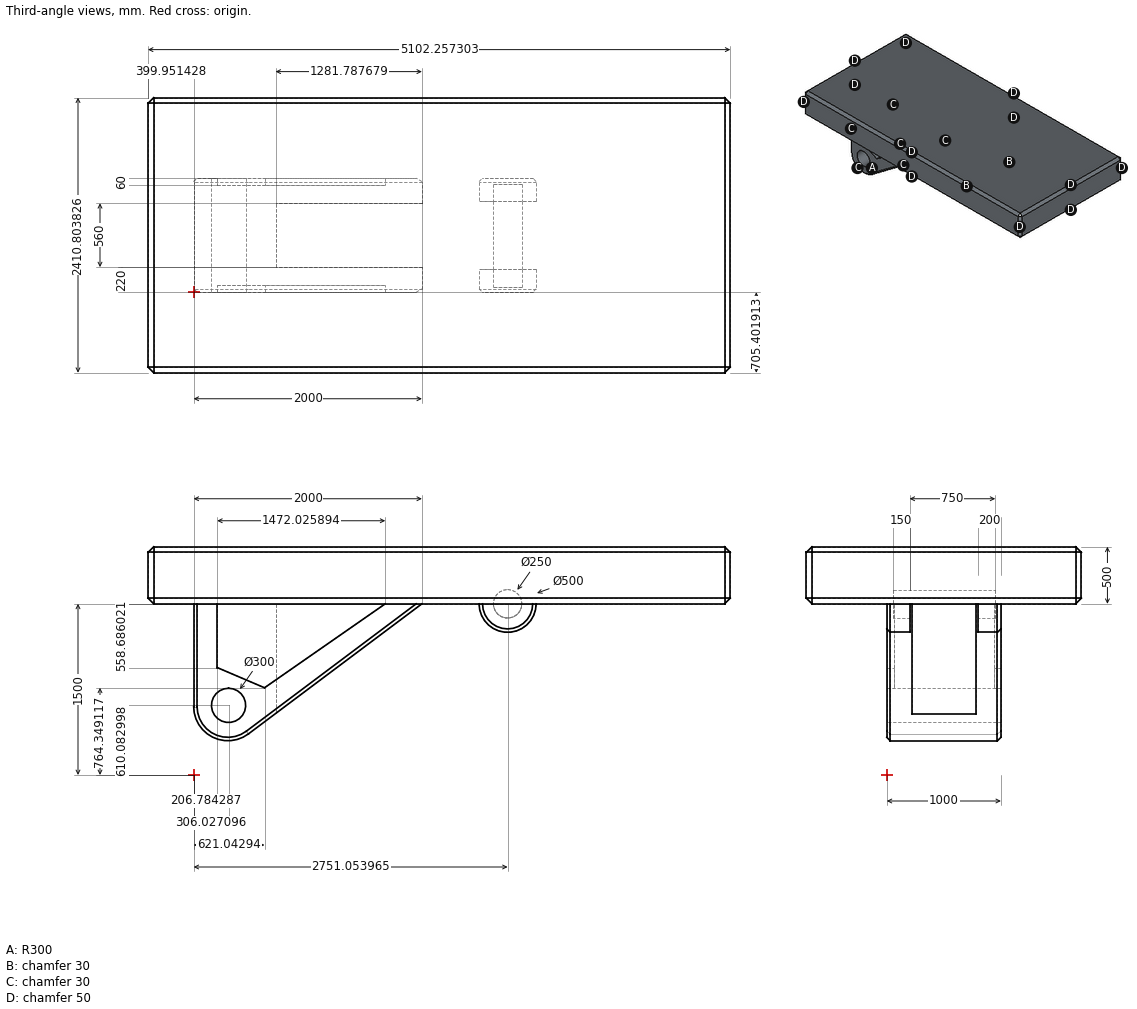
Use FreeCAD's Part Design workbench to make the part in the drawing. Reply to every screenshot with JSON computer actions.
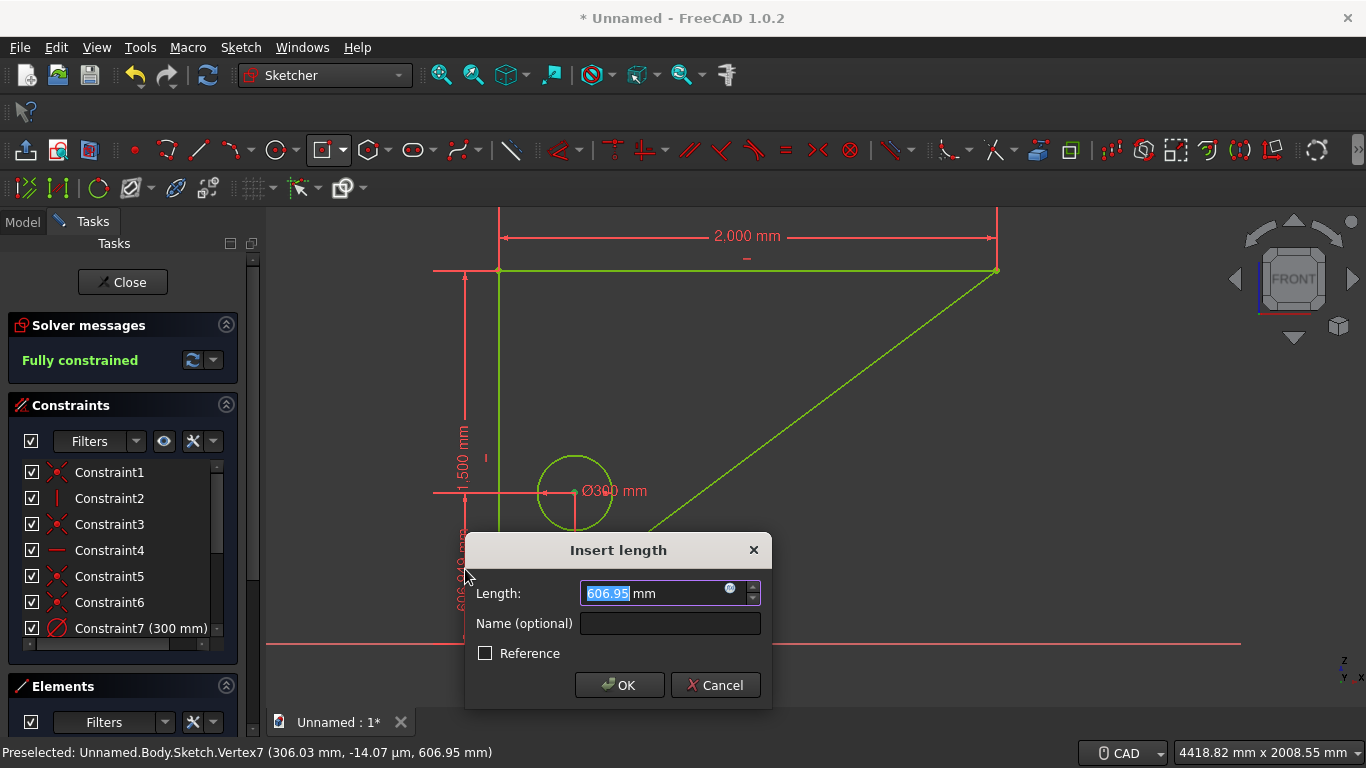
{"action": "type", "text": "610.082998"}
{"action": "key", "text": "Return"}
{"action": "key", "text": "Escape"}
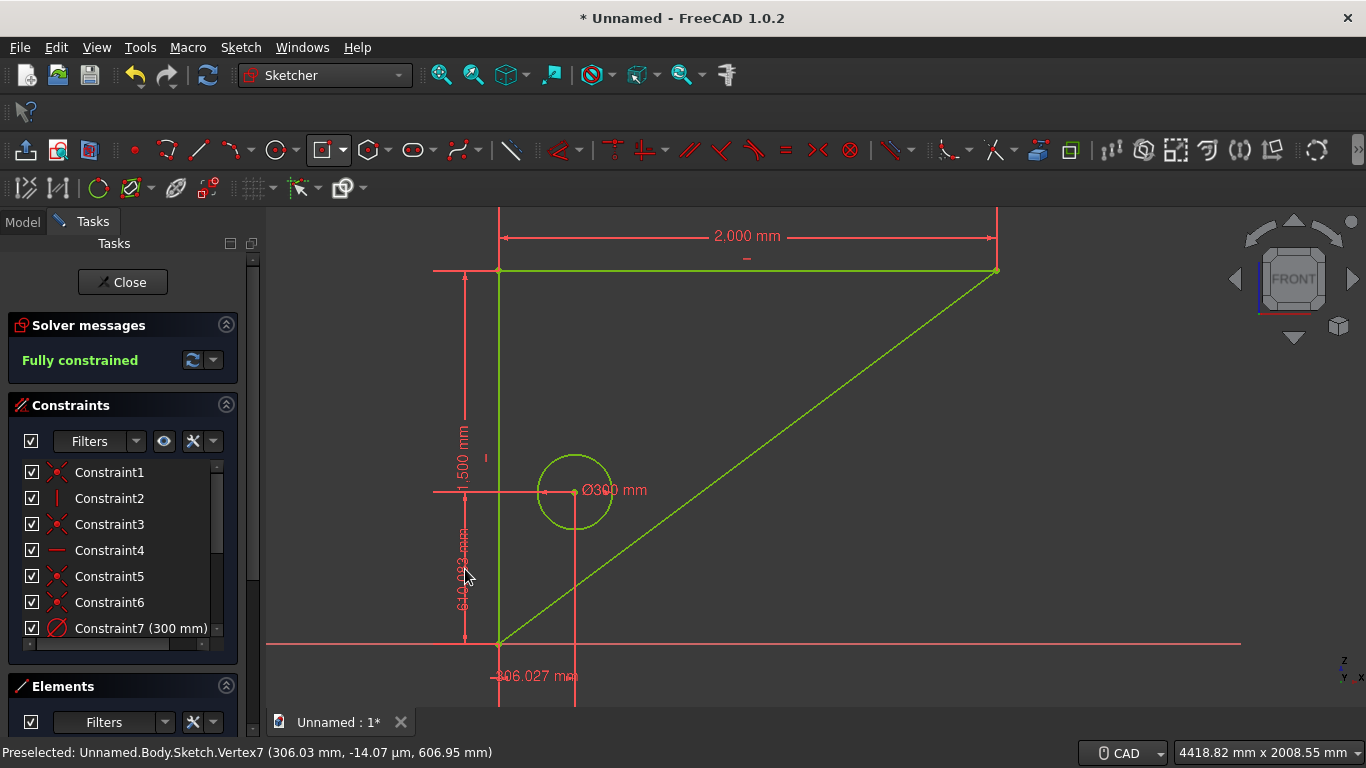
{"action": "left_click", "coordinate": [123, 282]}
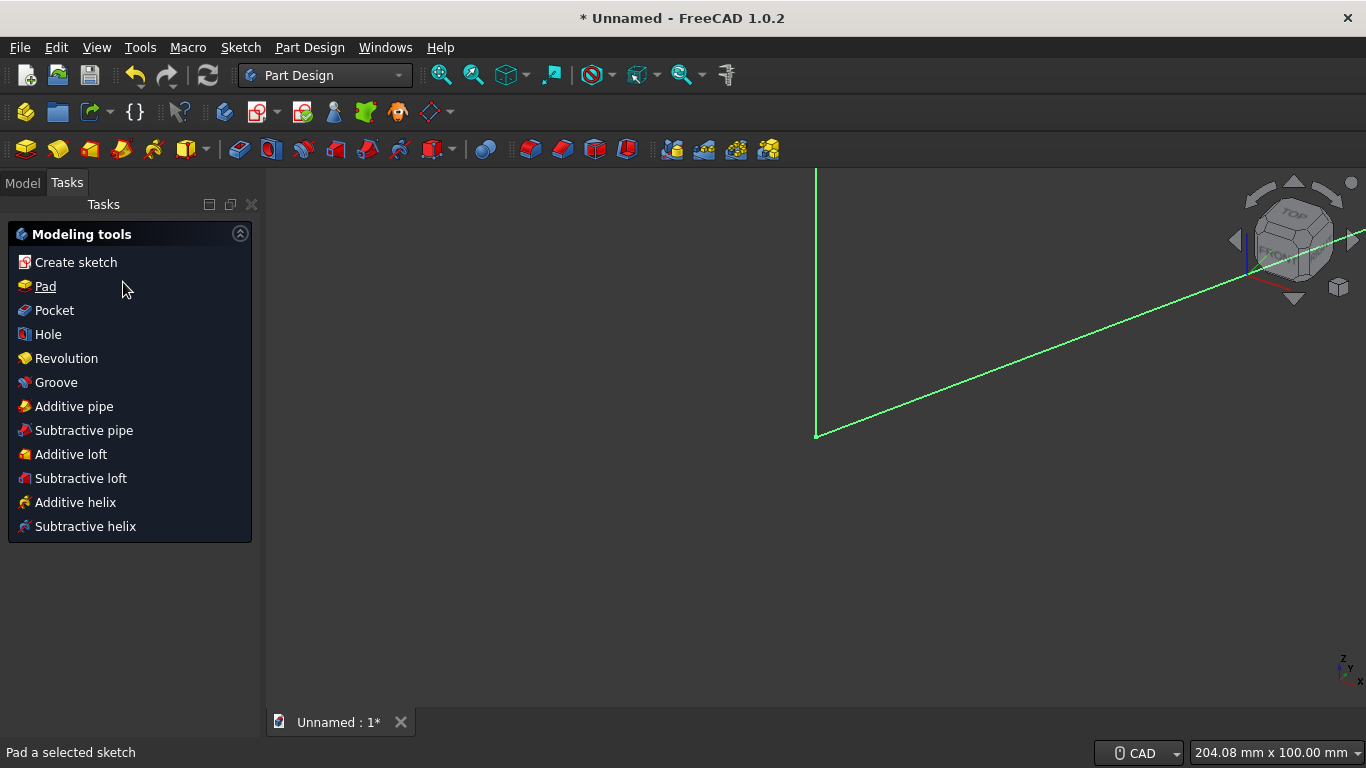
{"action": "left_click", "coordinate": [26, 150]}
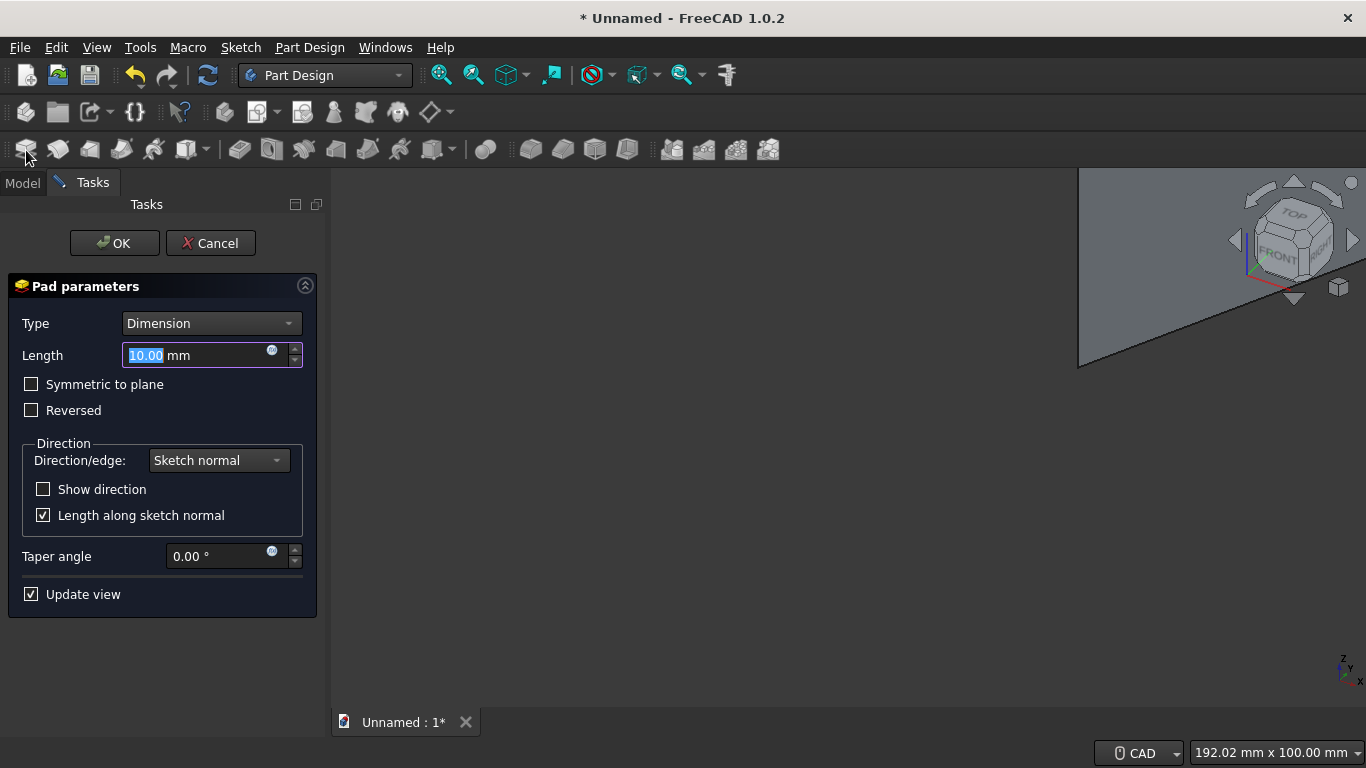
{"action": "type", "text": "1000"}
{"action": "key", "text": "Tab"}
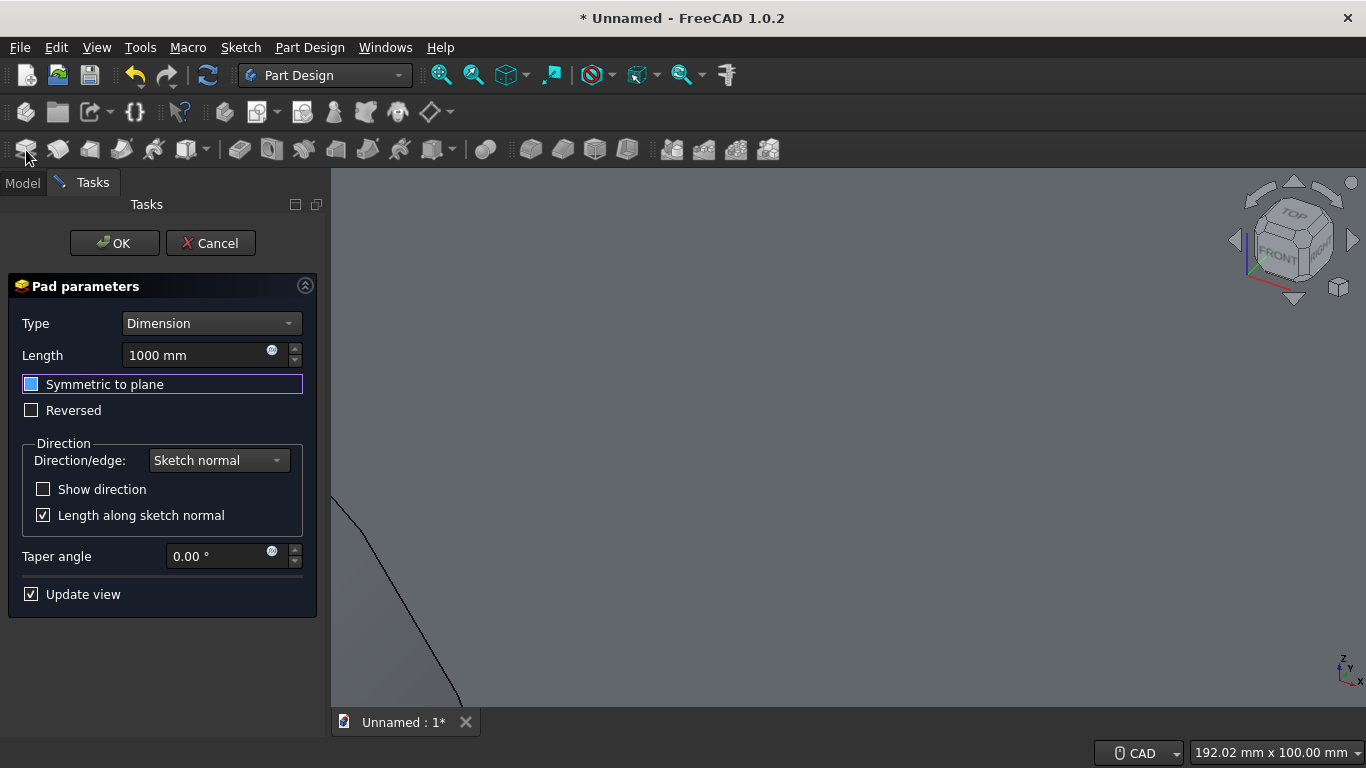
{"action": "left_click", "coordinate": [30, 410]}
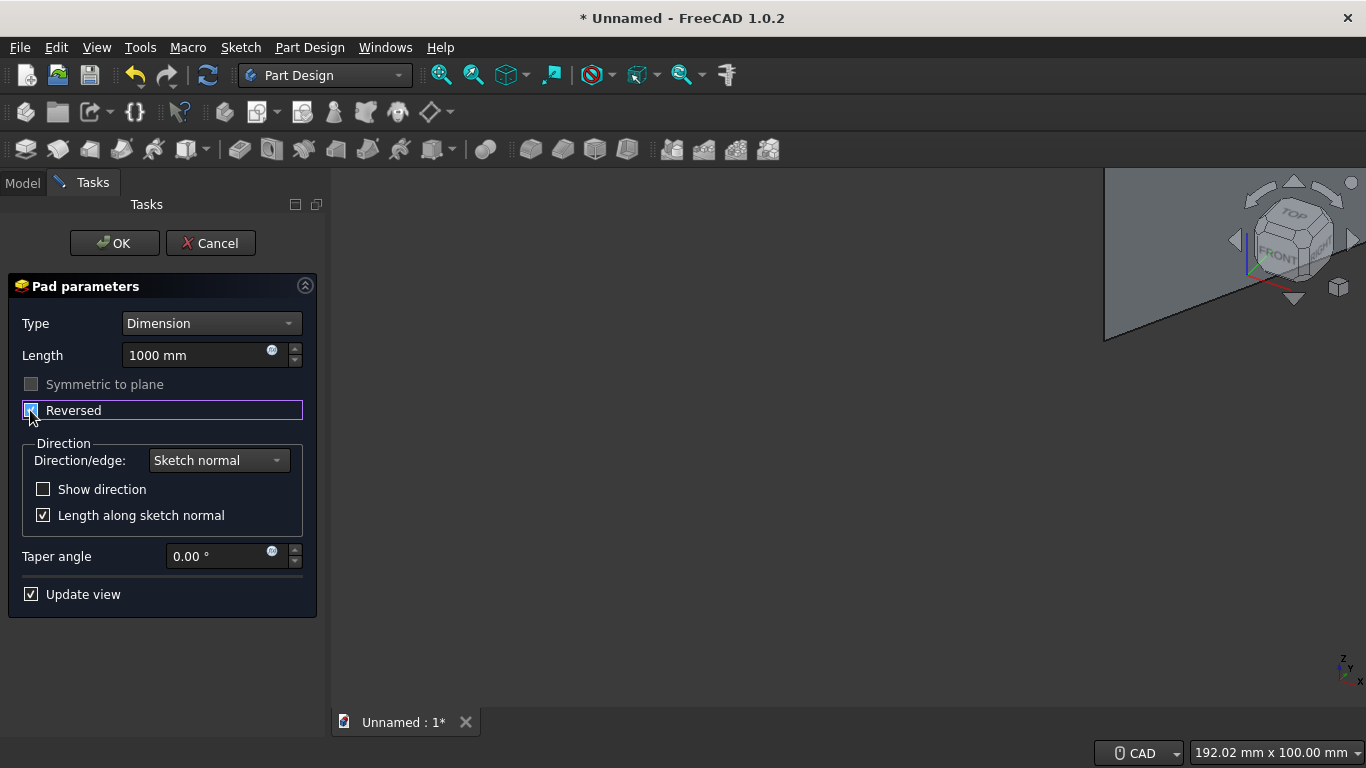
{"action": "left_click", "coordinate": [115, 243]}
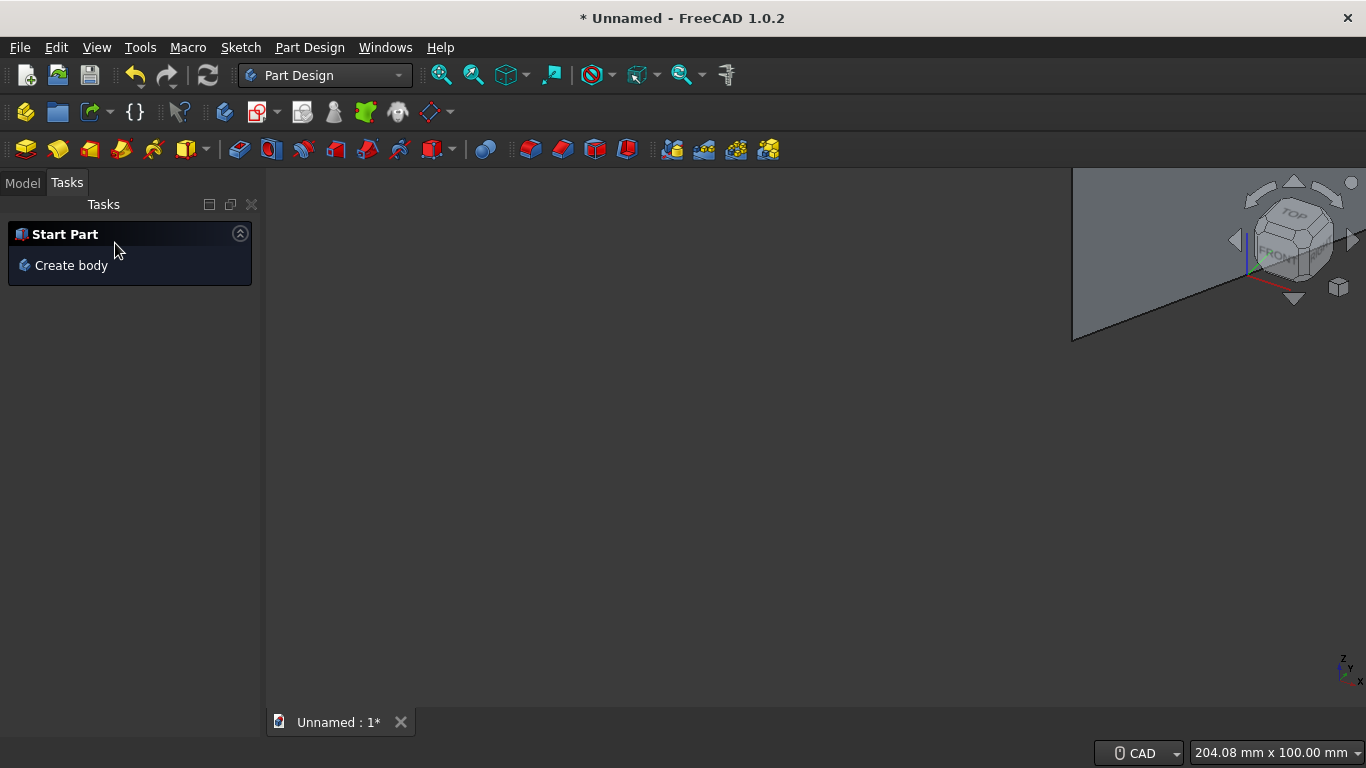
{"action": "left_click", "coordinate": [442, 76]}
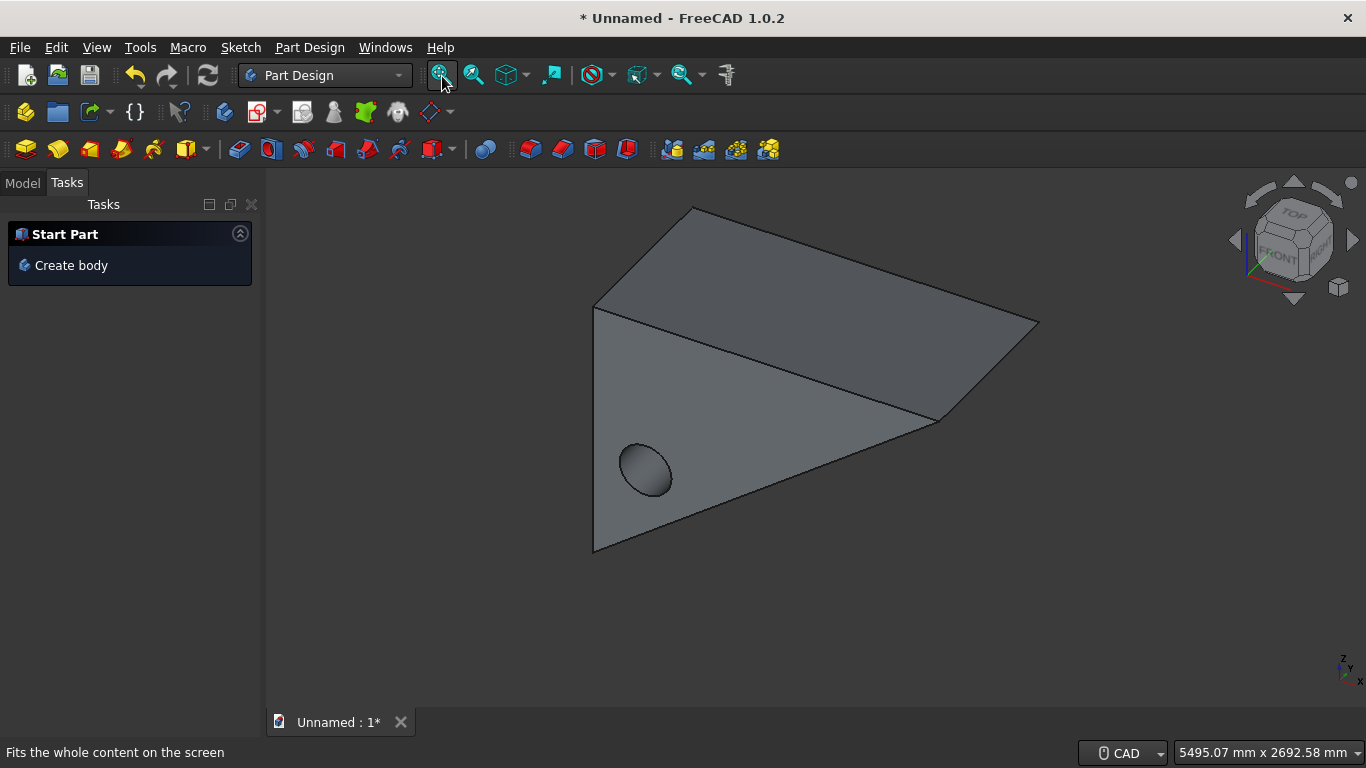
{"action": "key", "text": "0"}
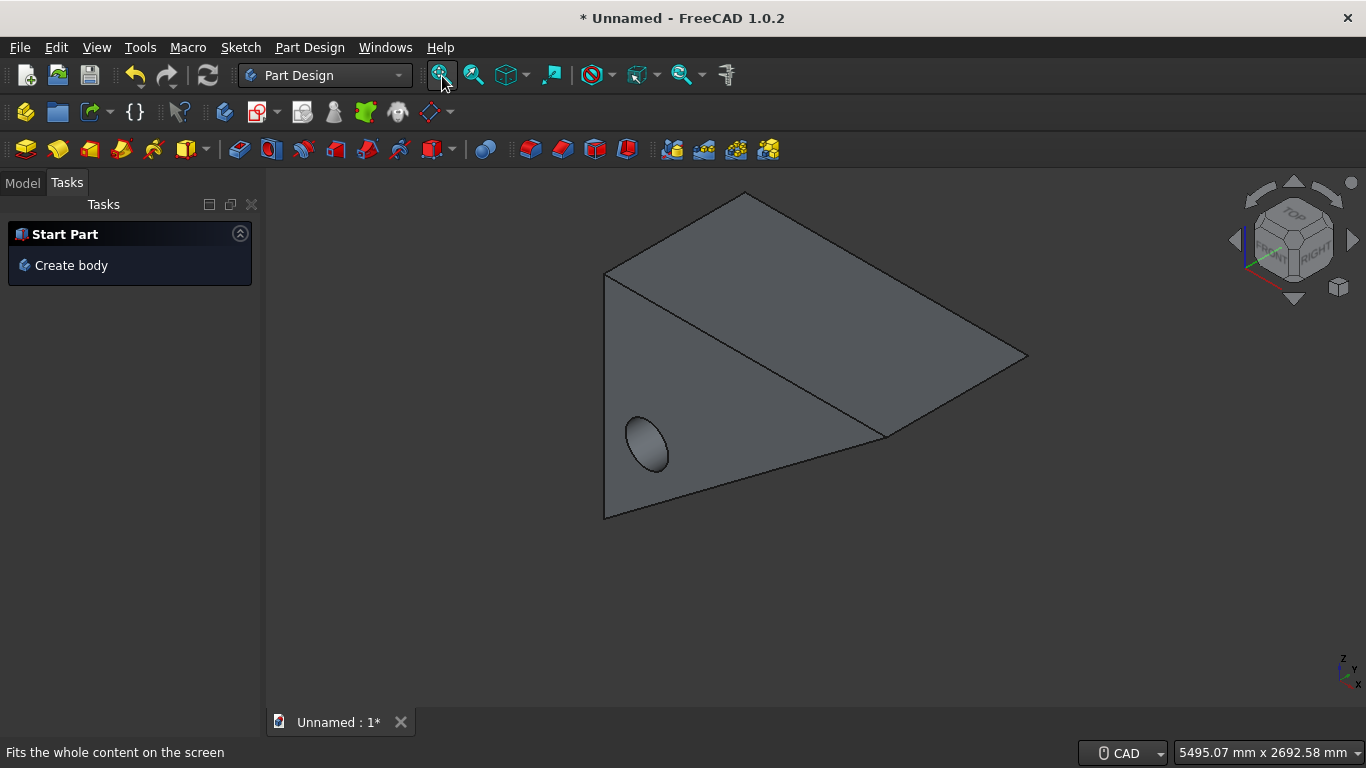
{"action": "key", "text": "2"}